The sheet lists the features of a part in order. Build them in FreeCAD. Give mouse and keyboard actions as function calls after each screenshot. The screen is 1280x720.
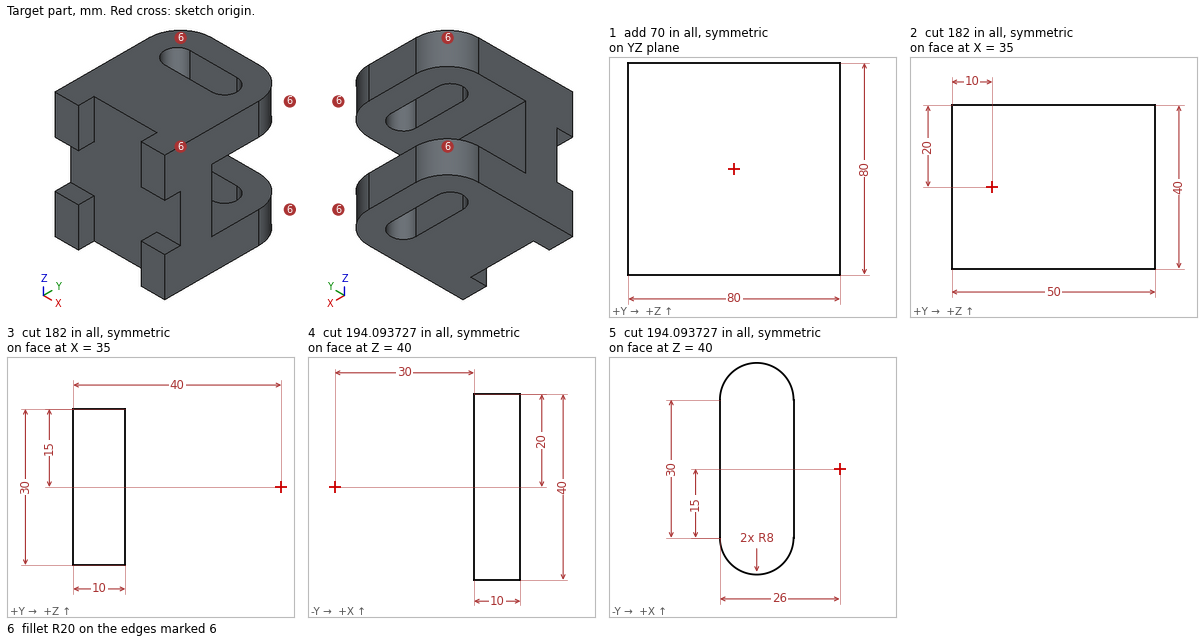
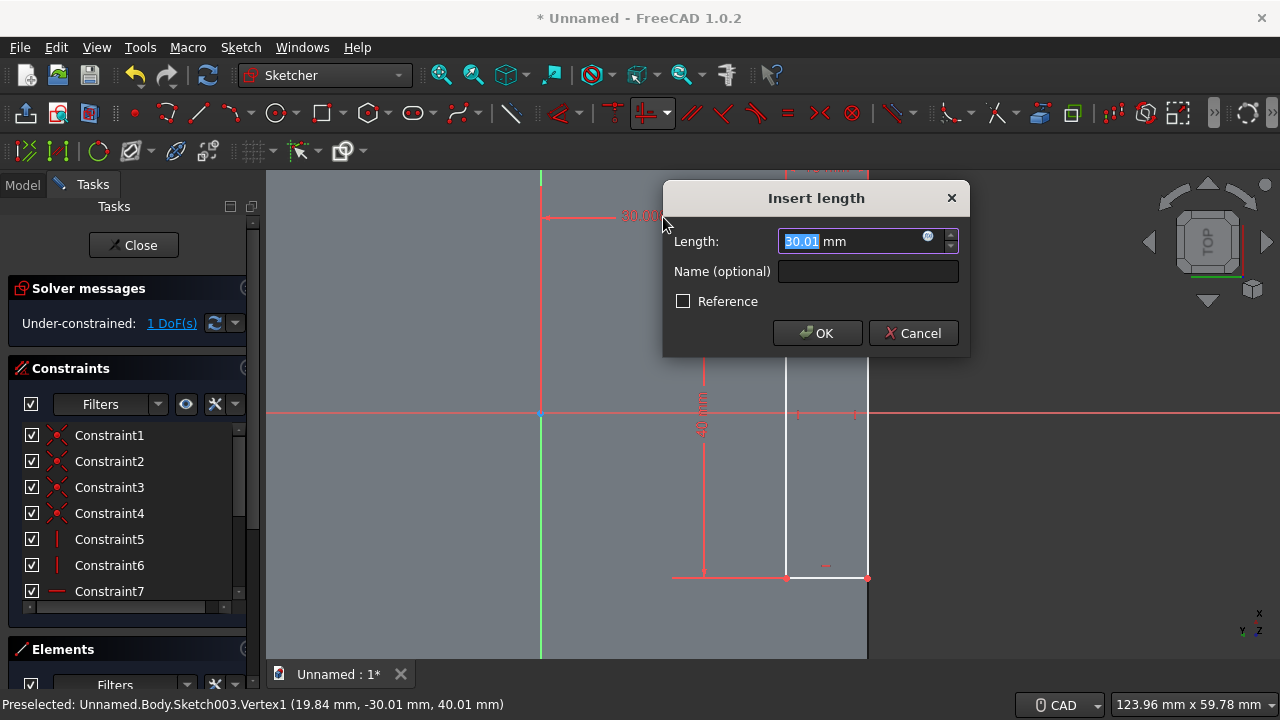
text(30)
key(Return)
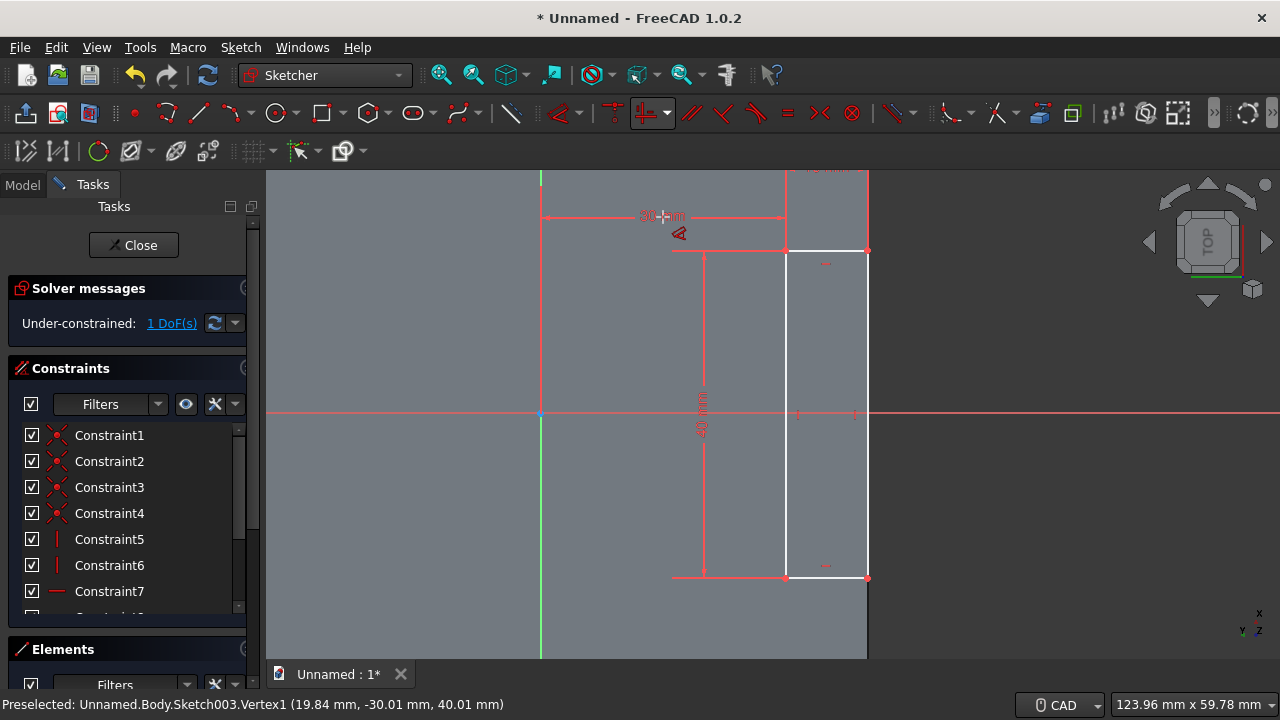
click(786, 251)
click(507, 332)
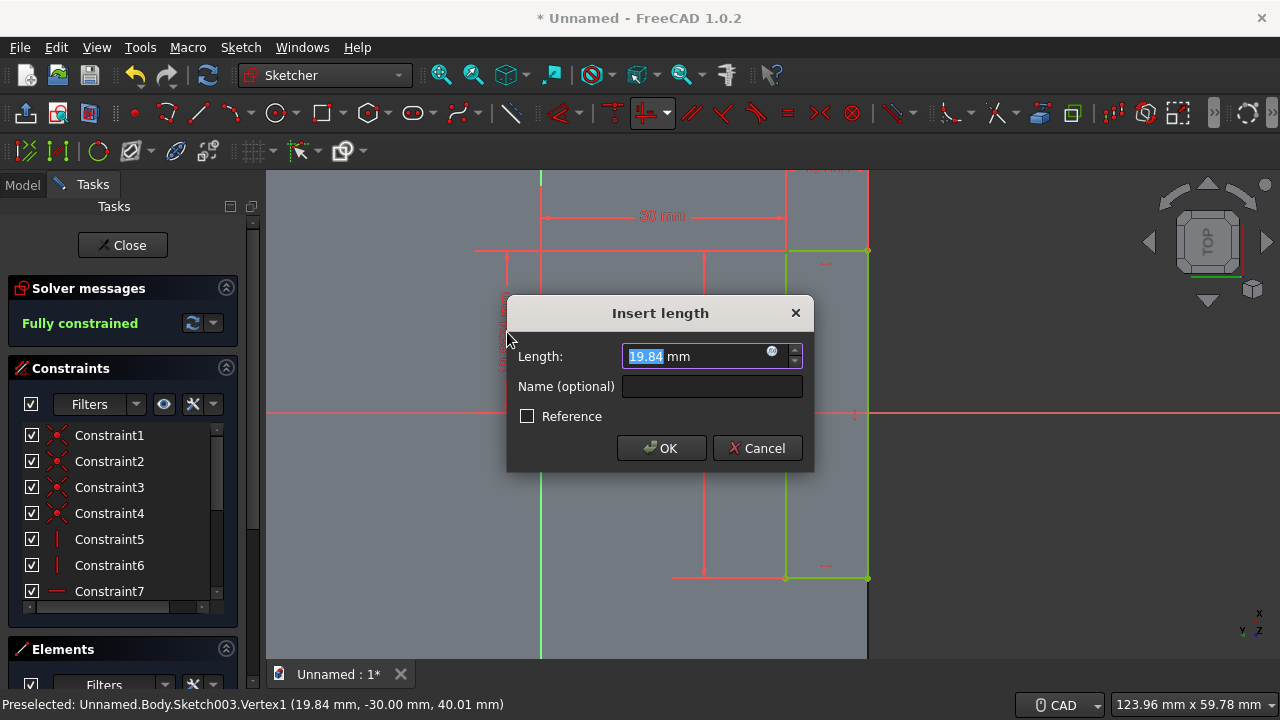
text(20)
key(Return)
key(Escape)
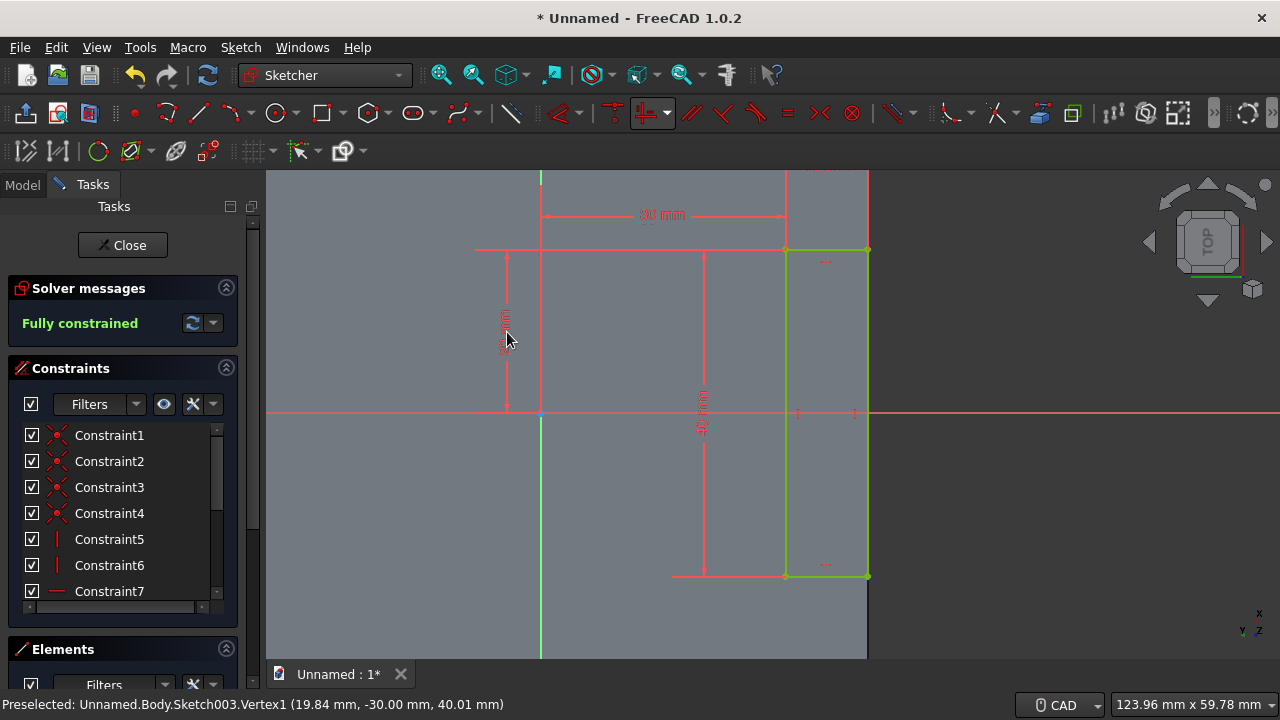
click(123, 245)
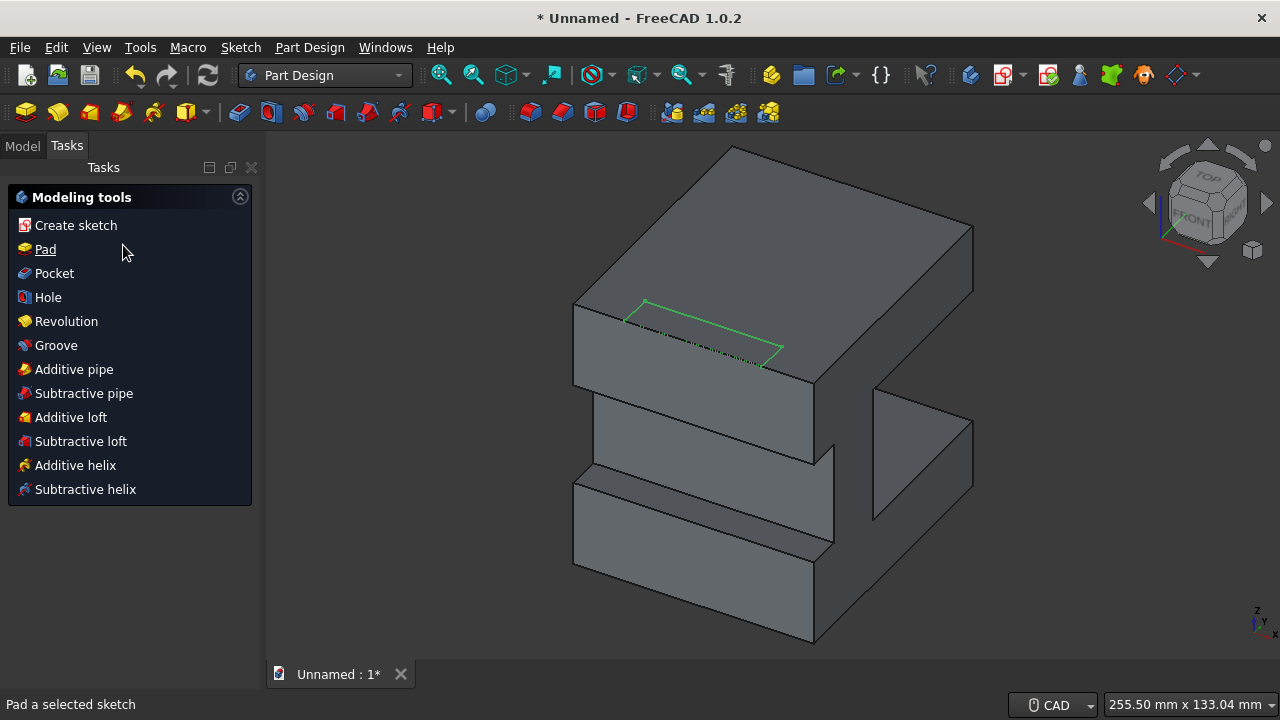
click(240, 112)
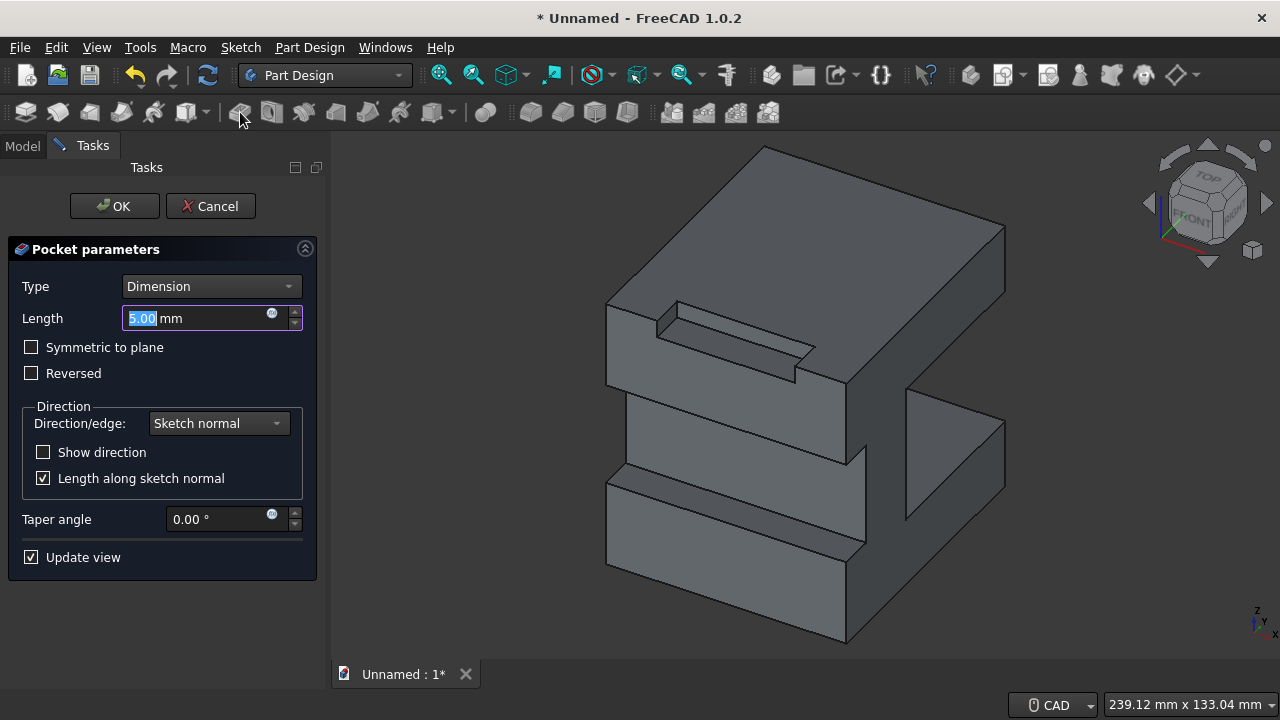
text(194.093727)
key(Tab)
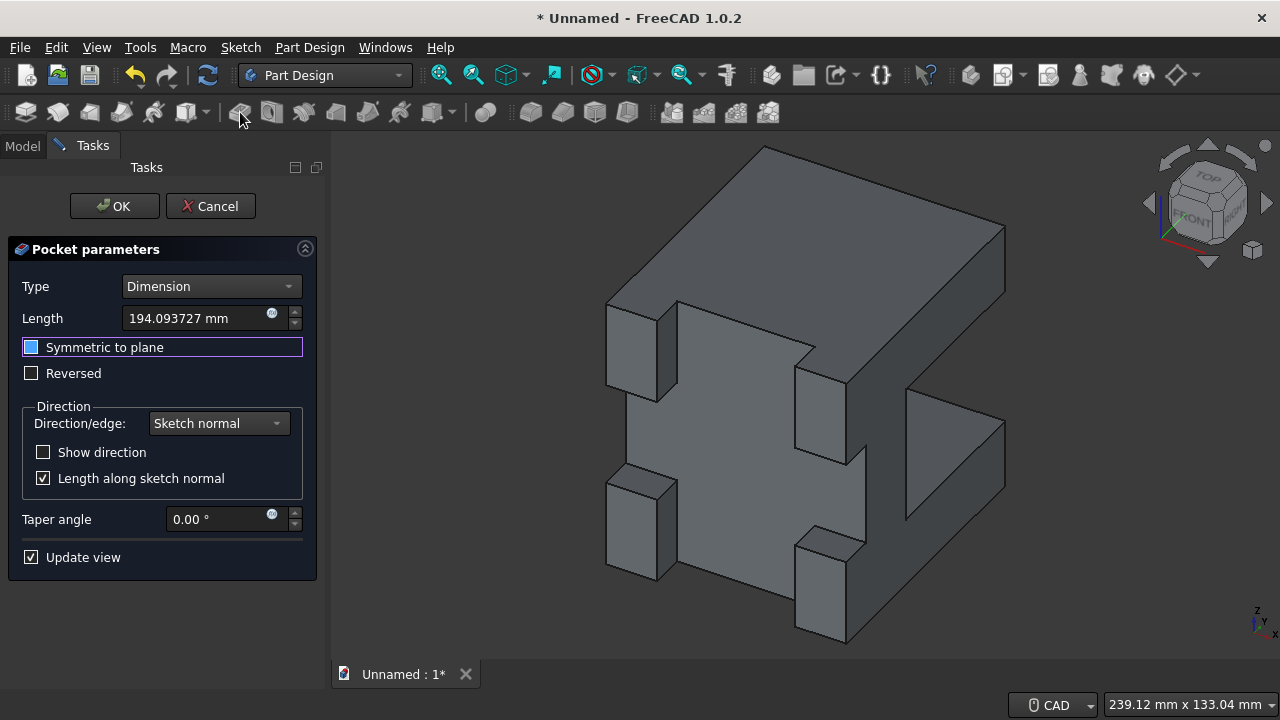
click(30, 347)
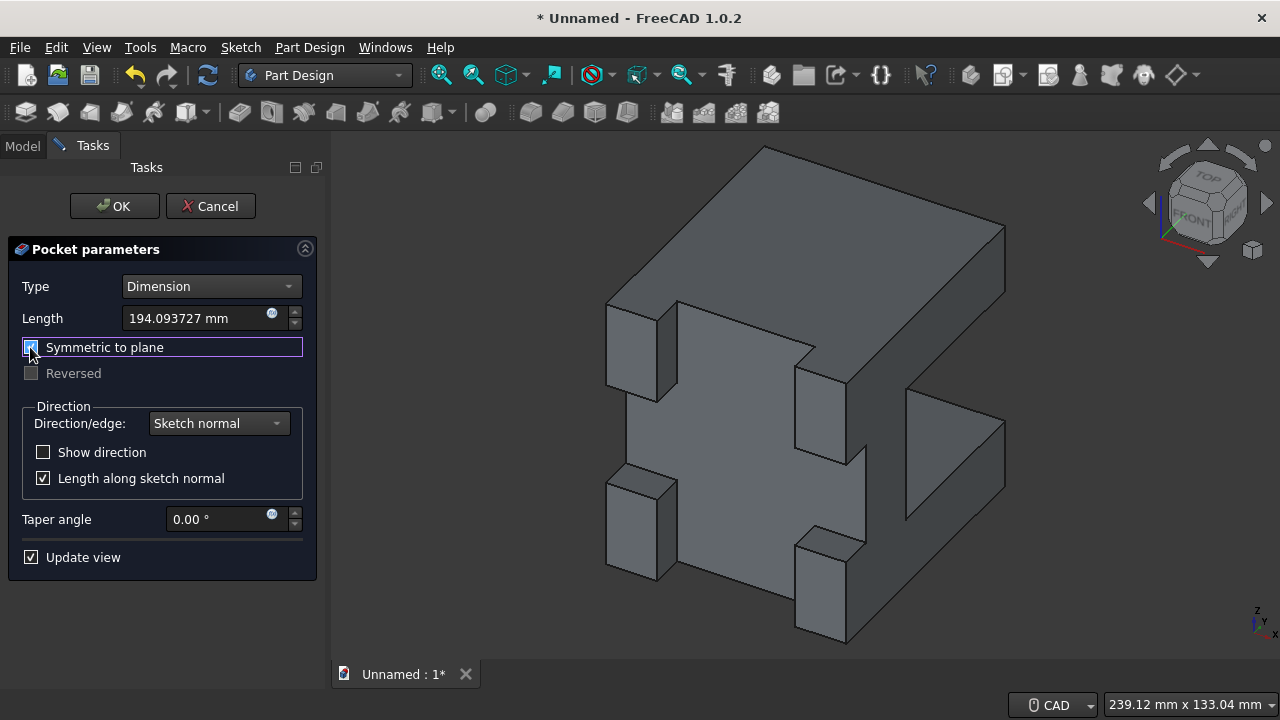
click(115, 206)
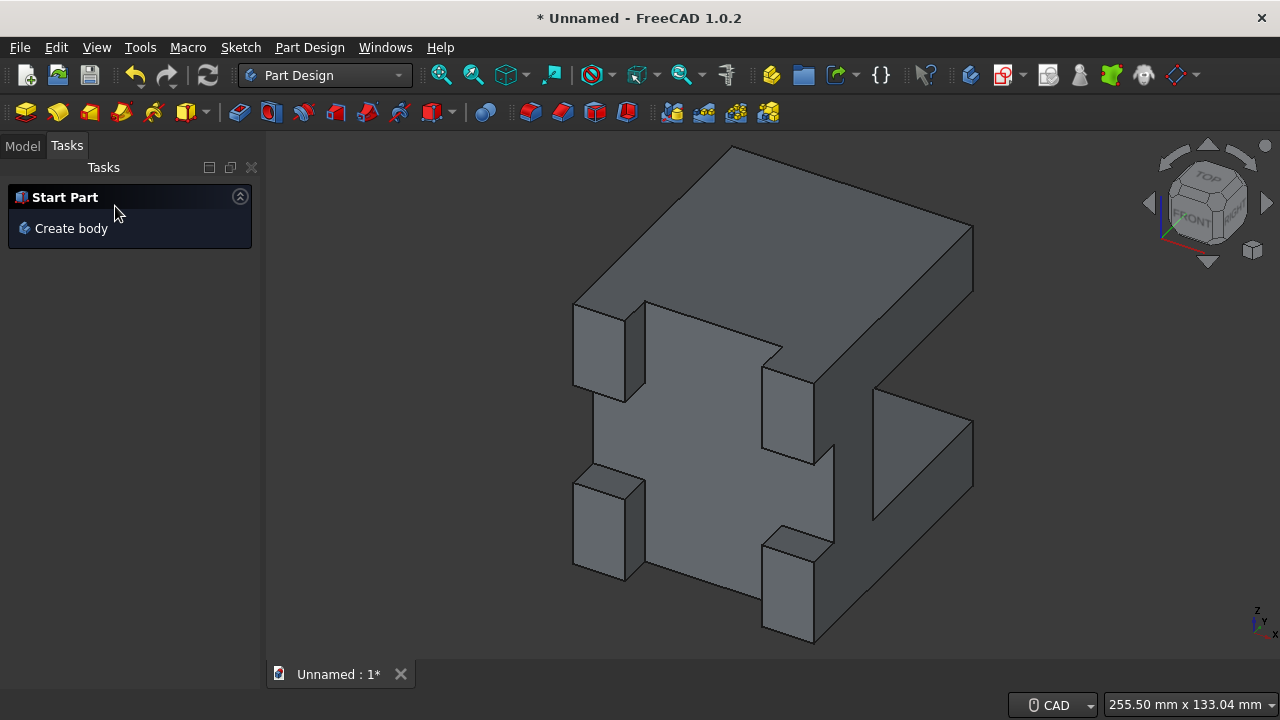
click(773, 264)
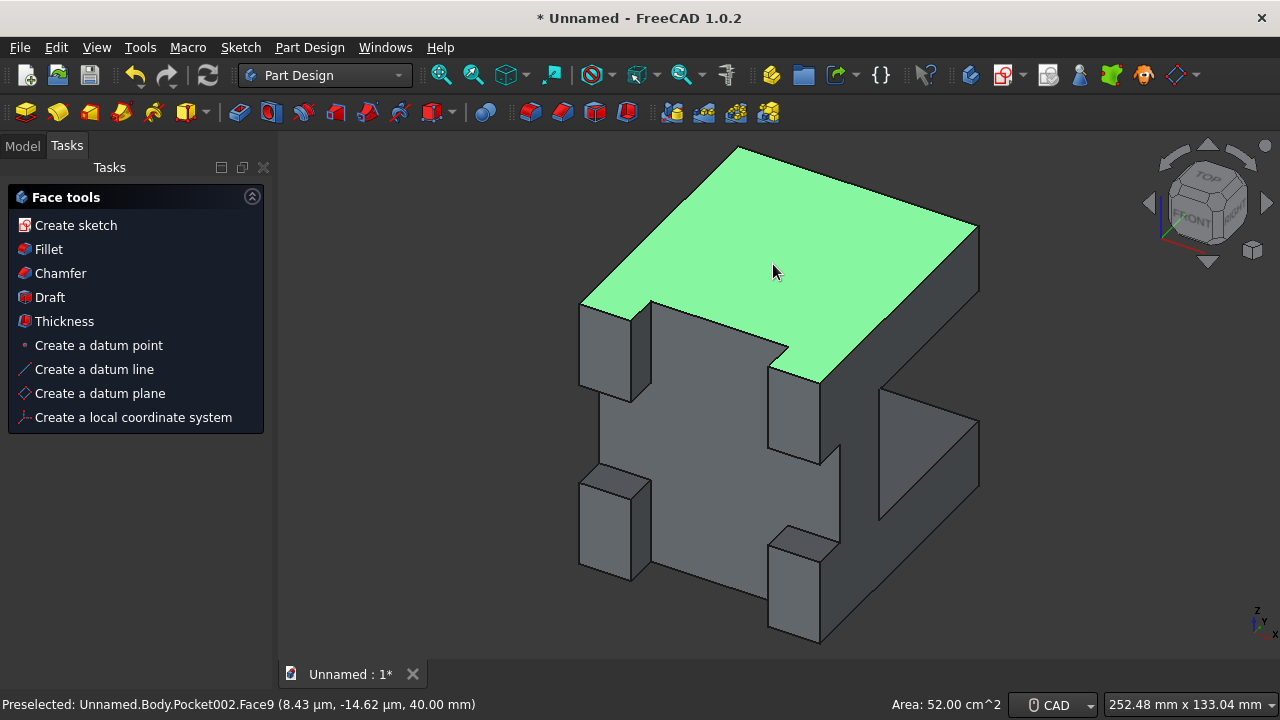
click(1004, 76)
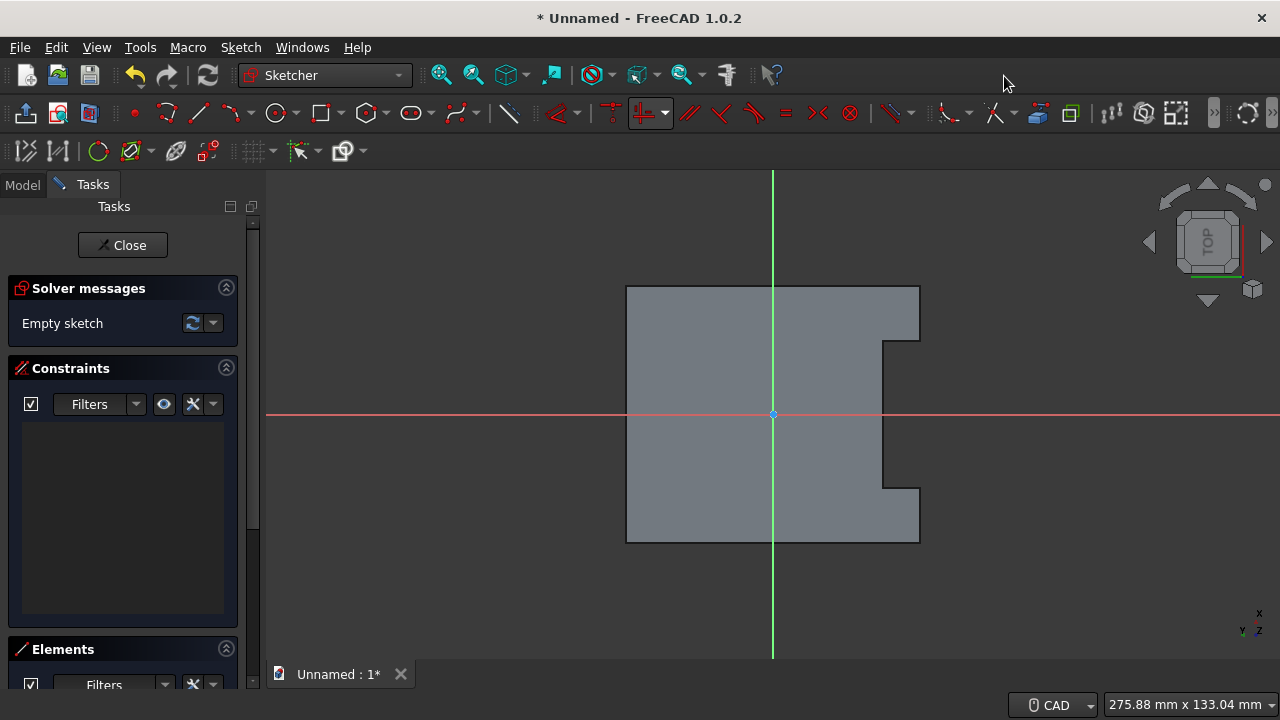
scroll(750, 415, up, 3)